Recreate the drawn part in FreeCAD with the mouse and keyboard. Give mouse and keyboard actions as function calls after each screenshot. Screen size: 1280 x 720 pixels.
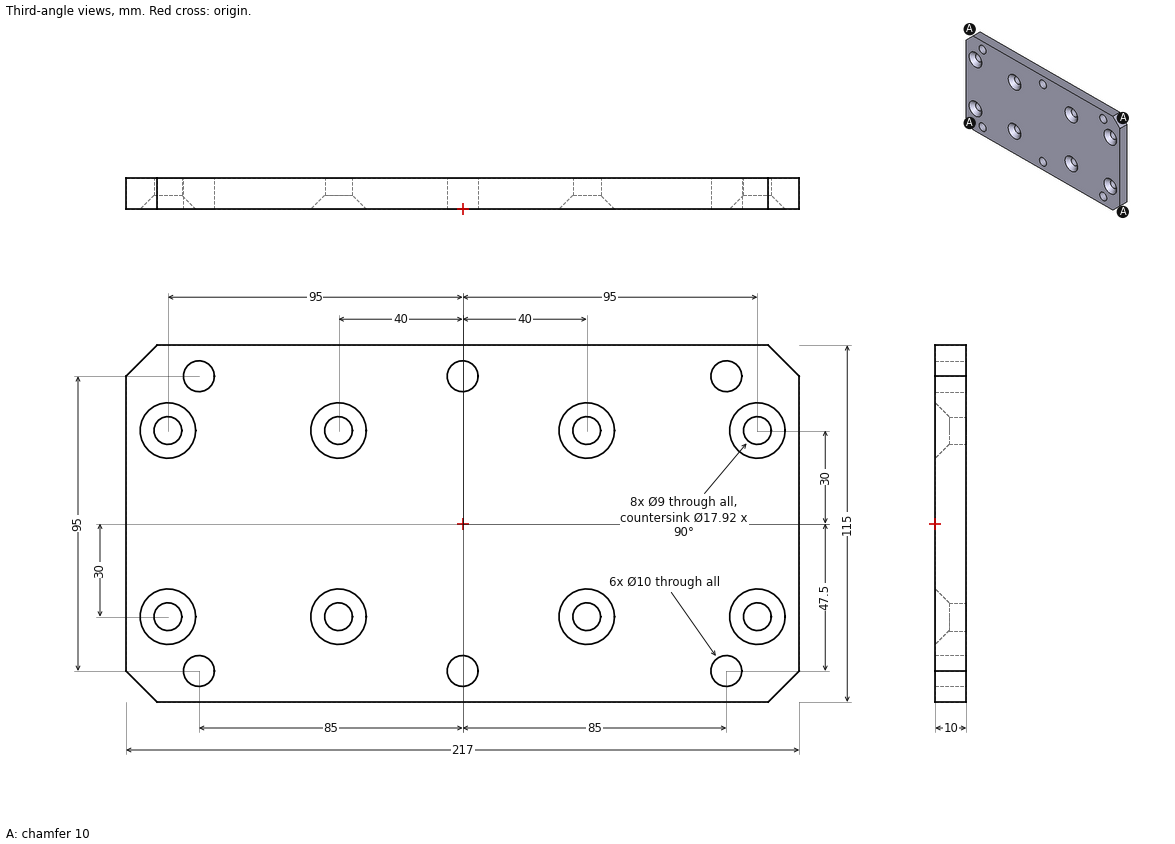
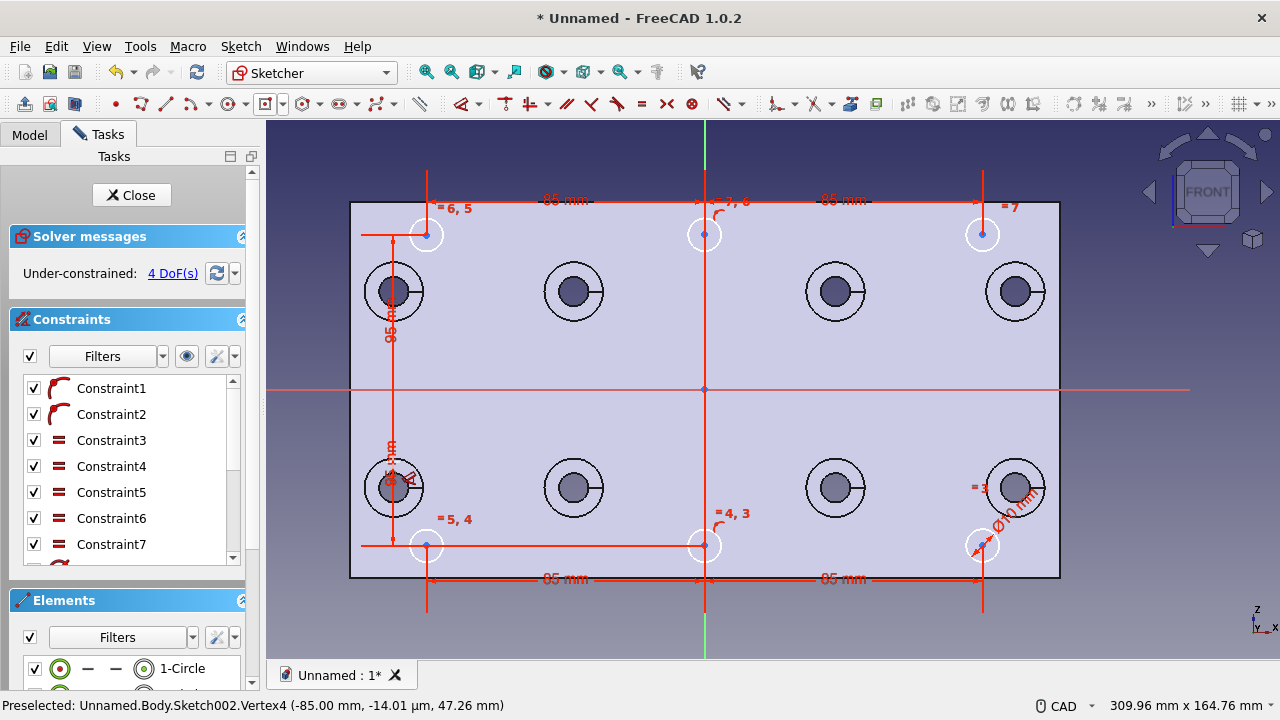
click(983, 546)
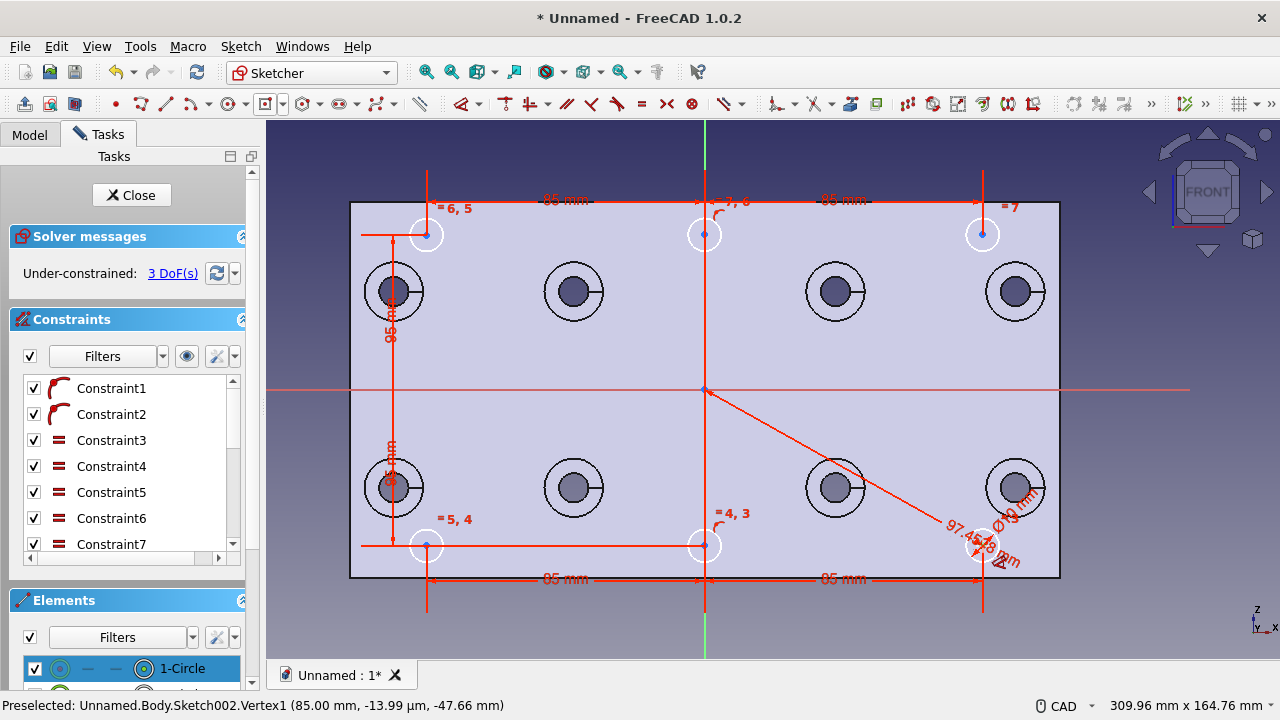
click(427, 235)
click(1017, 319)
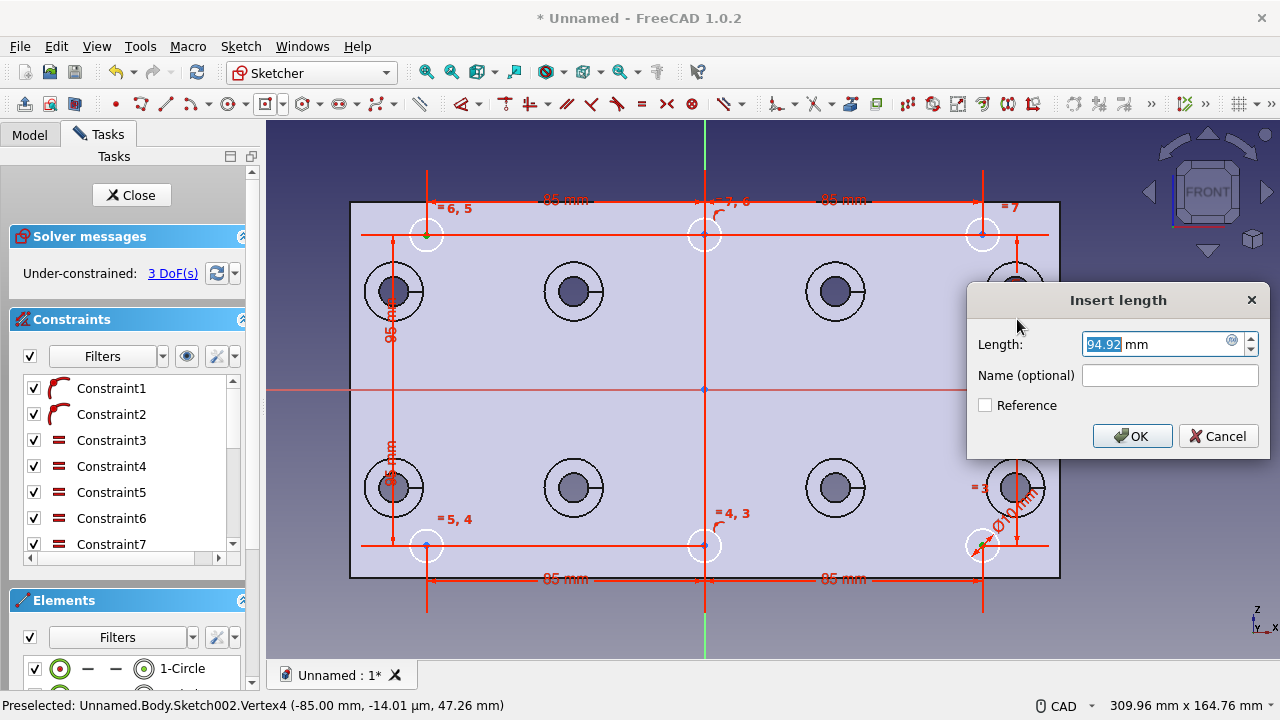
text(95)
key(Return)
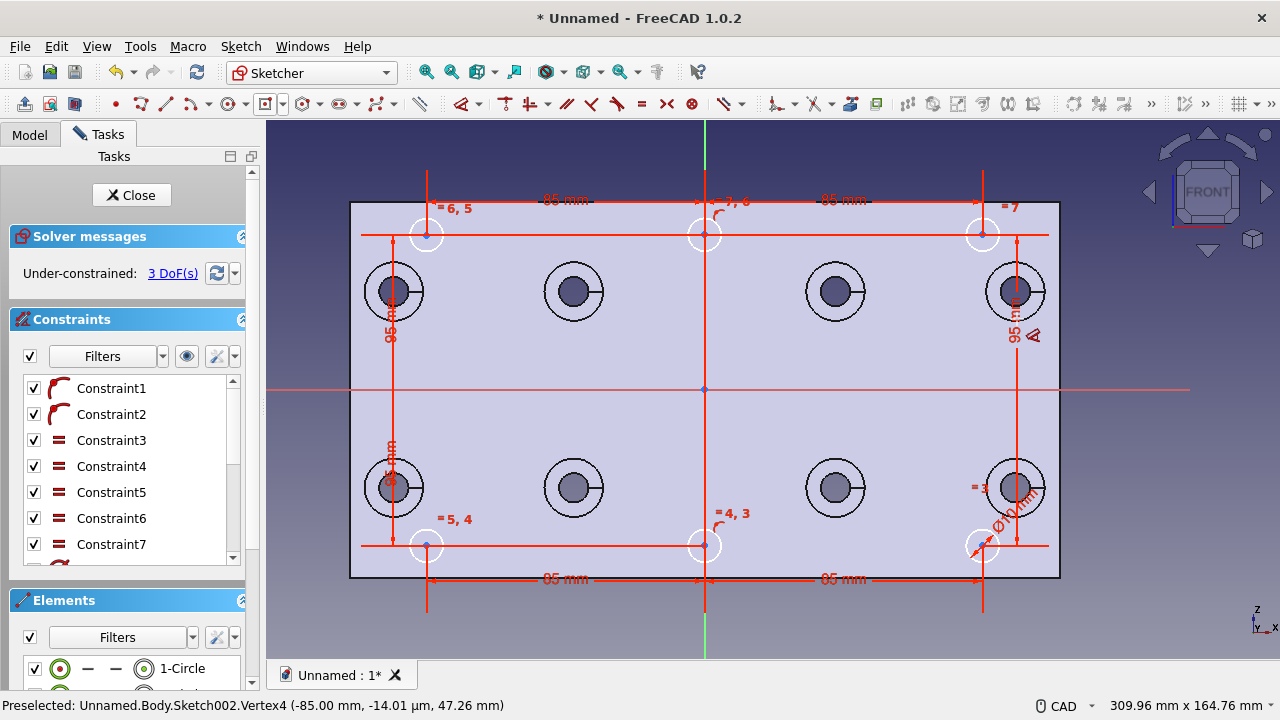
click(705, 546)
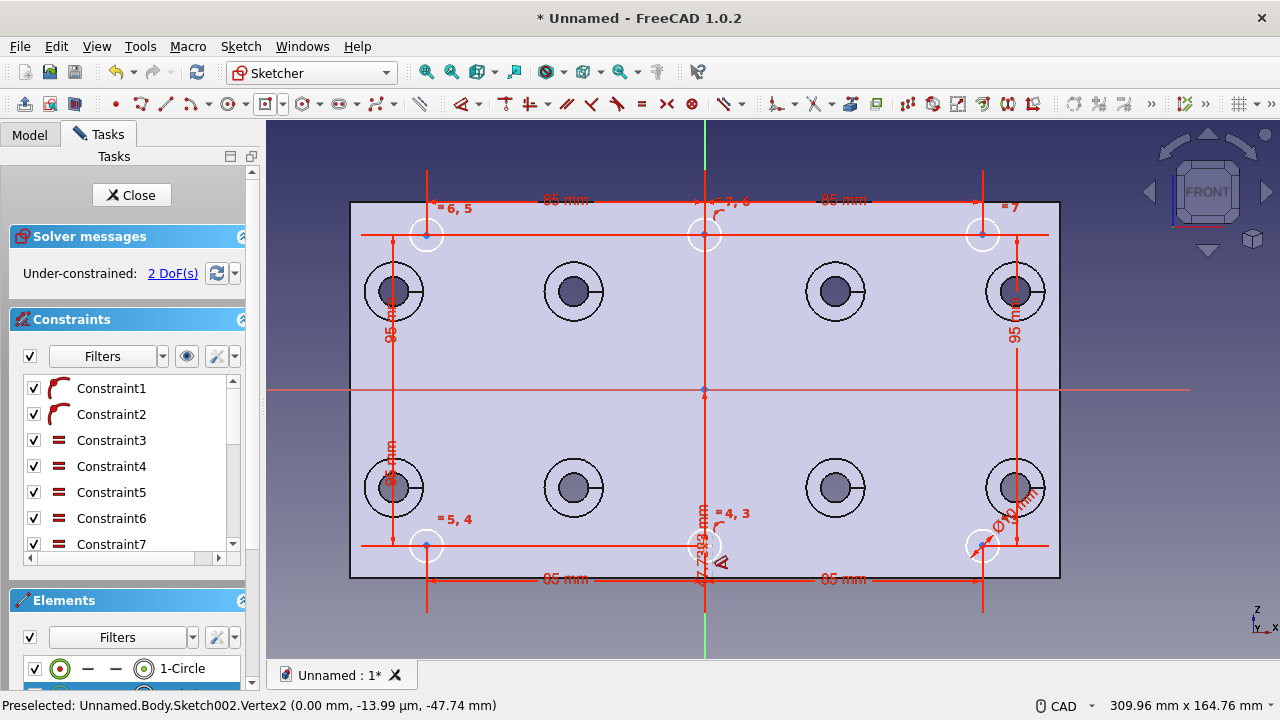
click(705, 235)
click(739, 319)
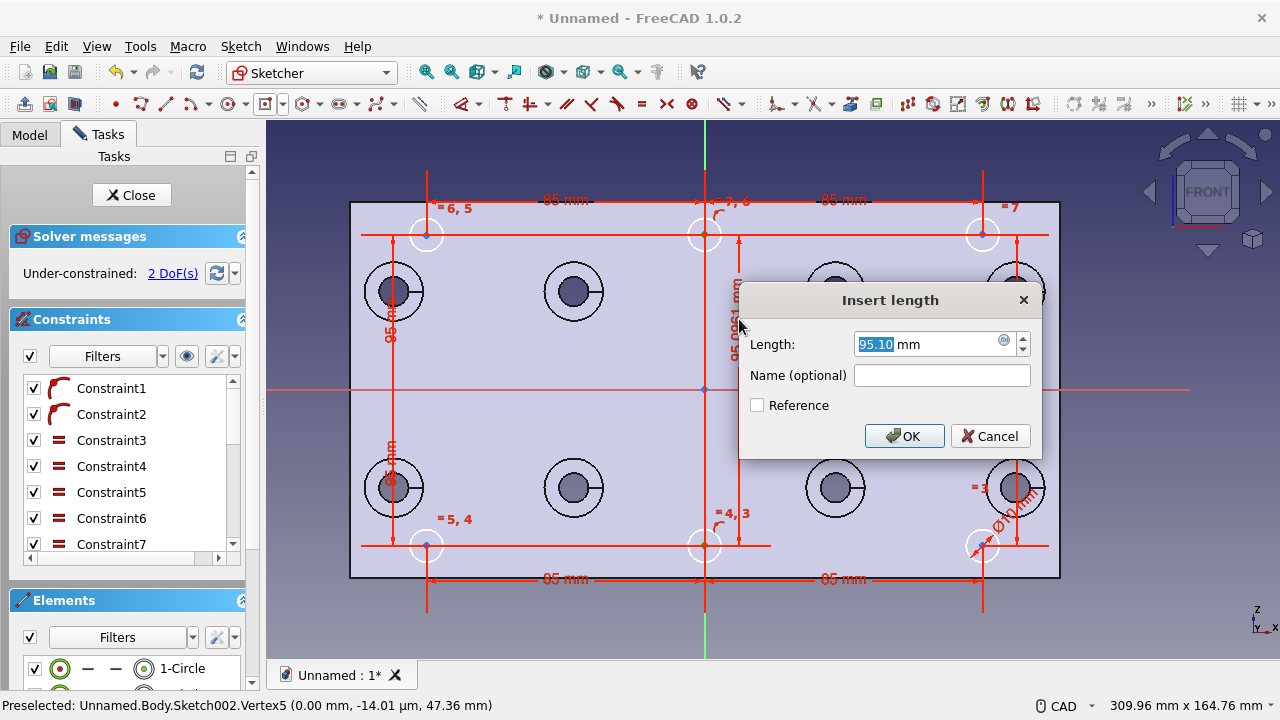
text(95)
key(Return)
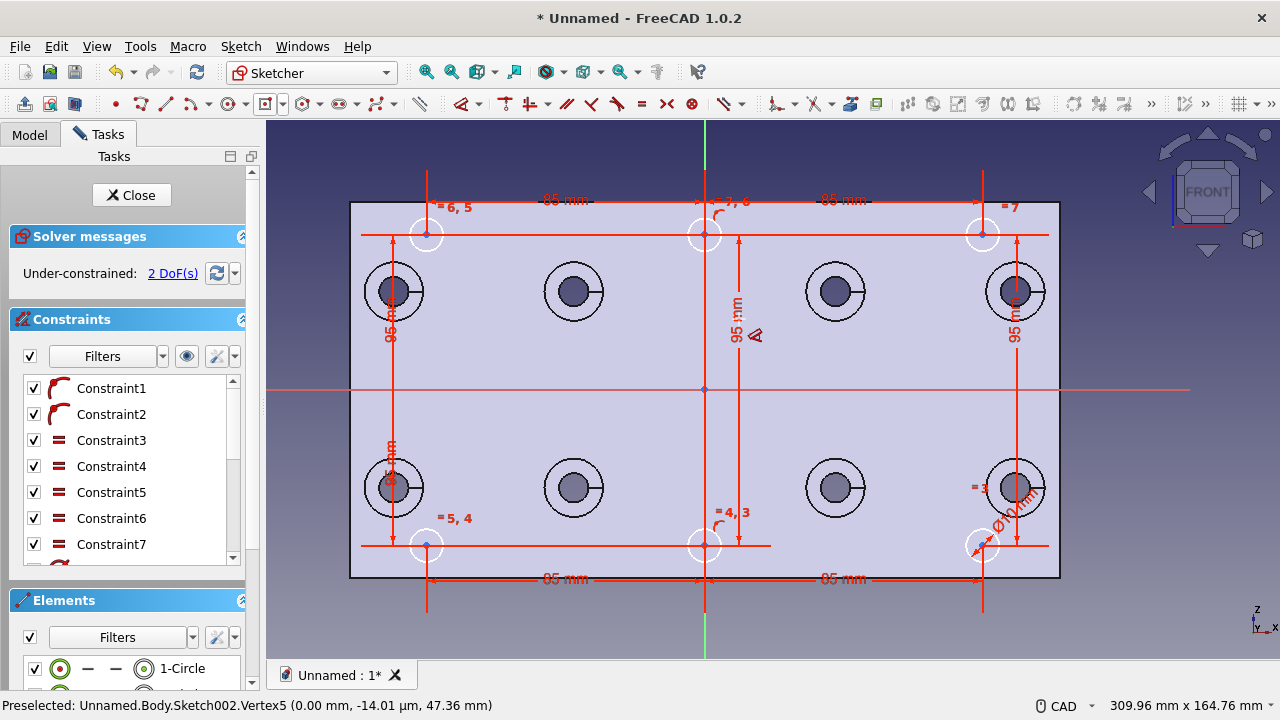
click(983, 546)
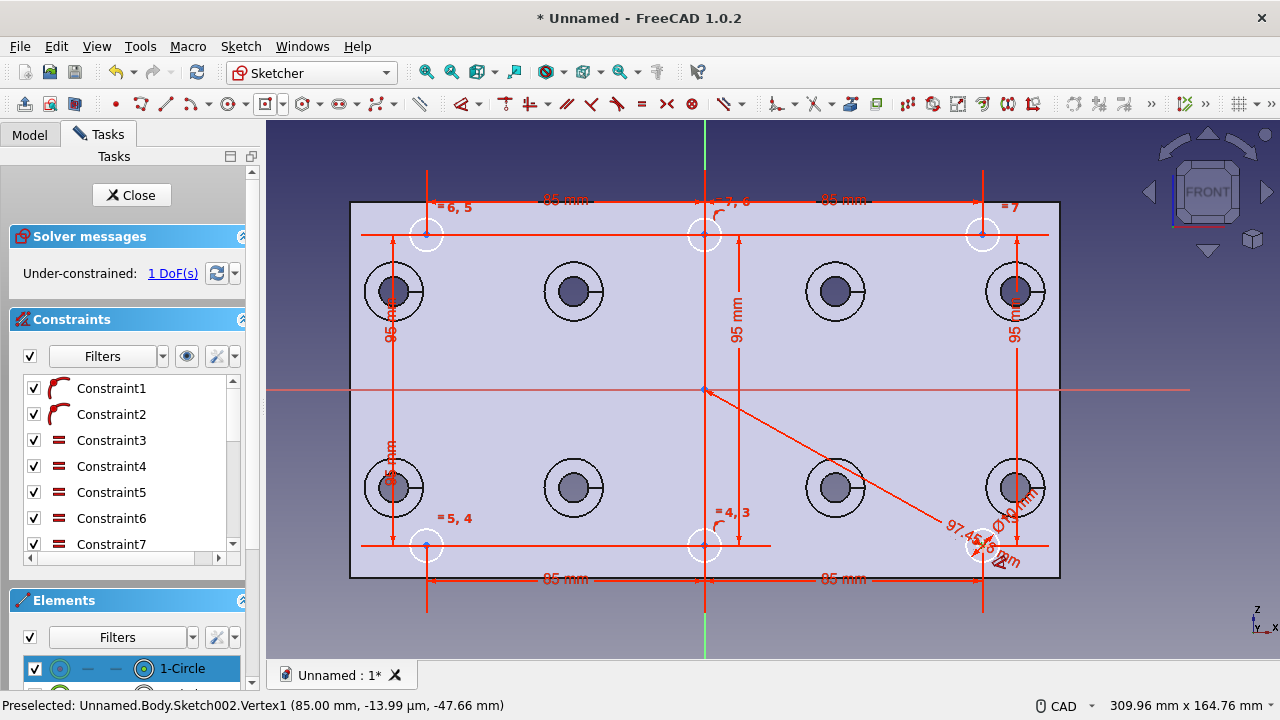
click(983, 235)
click(1017, 462)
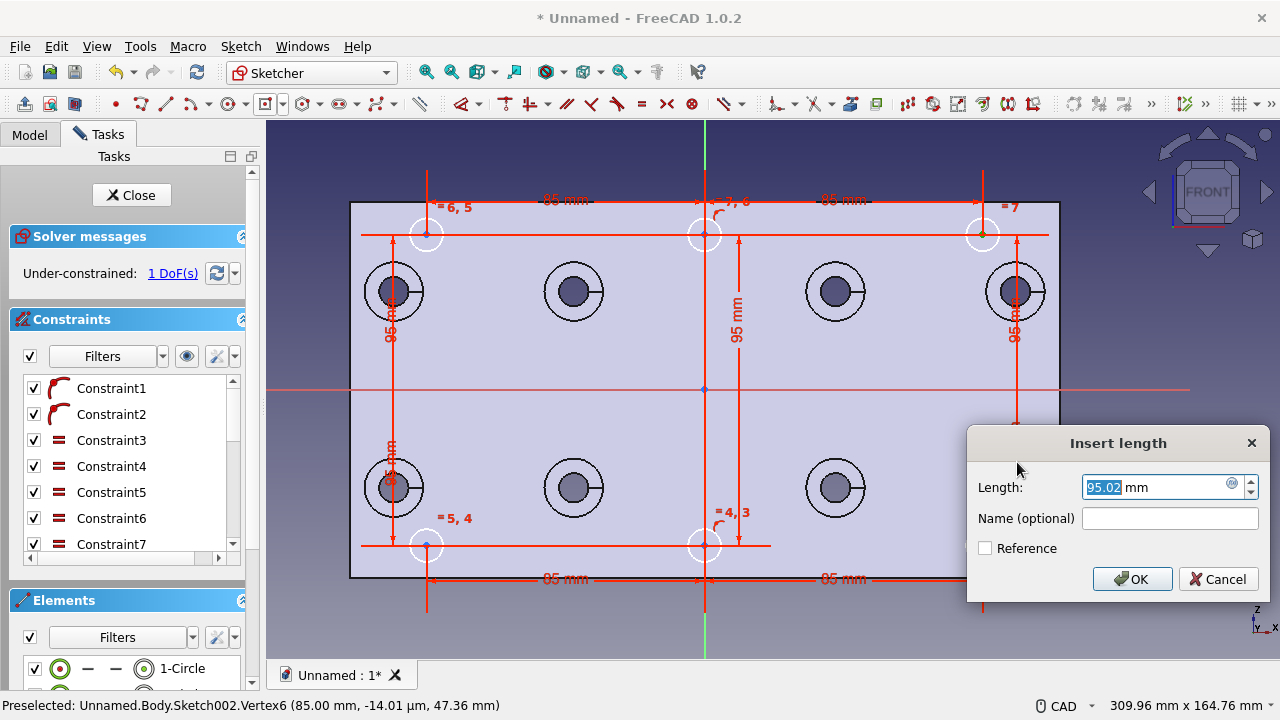
text(95)
key(Return)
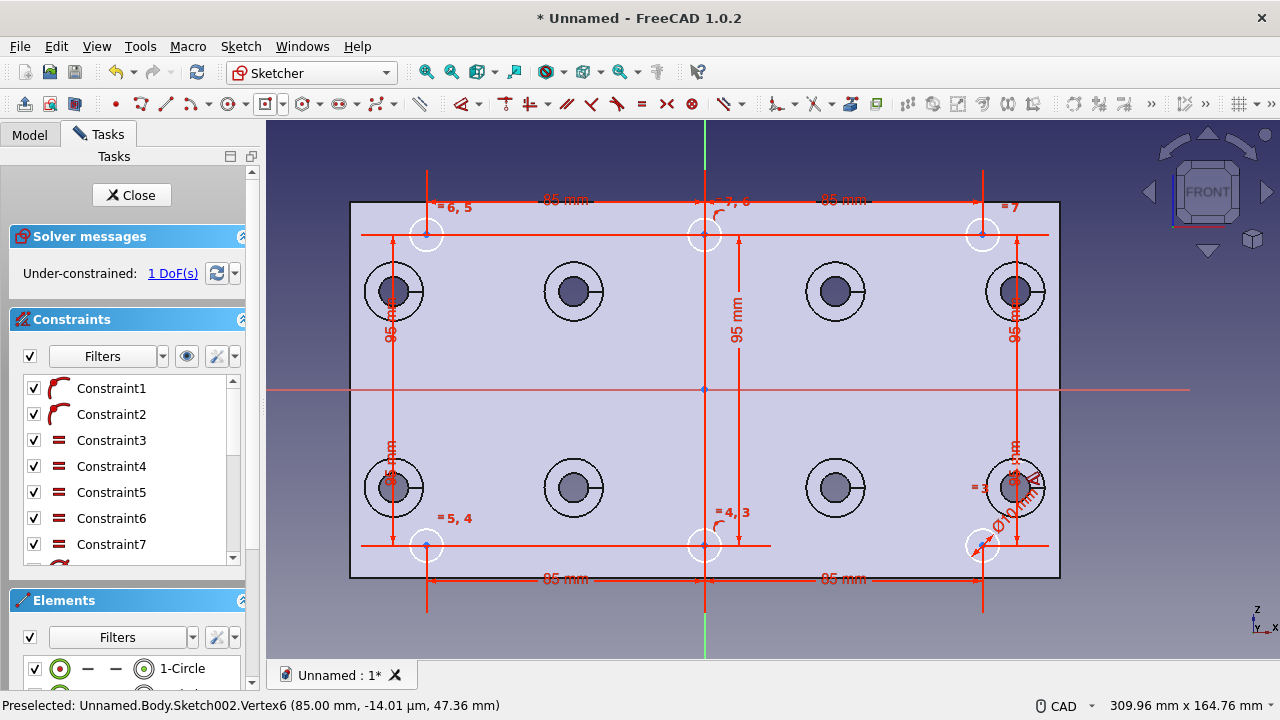
click(983, 546)
click(1017, 432)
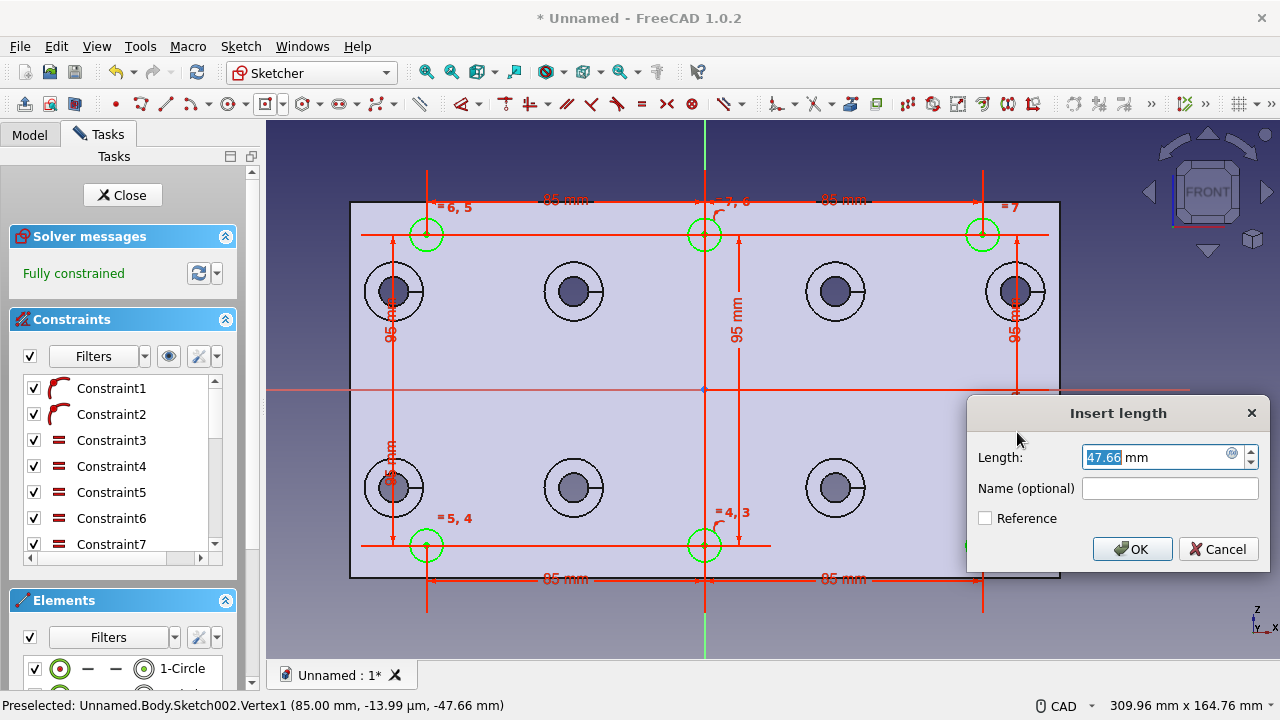
text(47.5)
key(Return)
key(Escape)